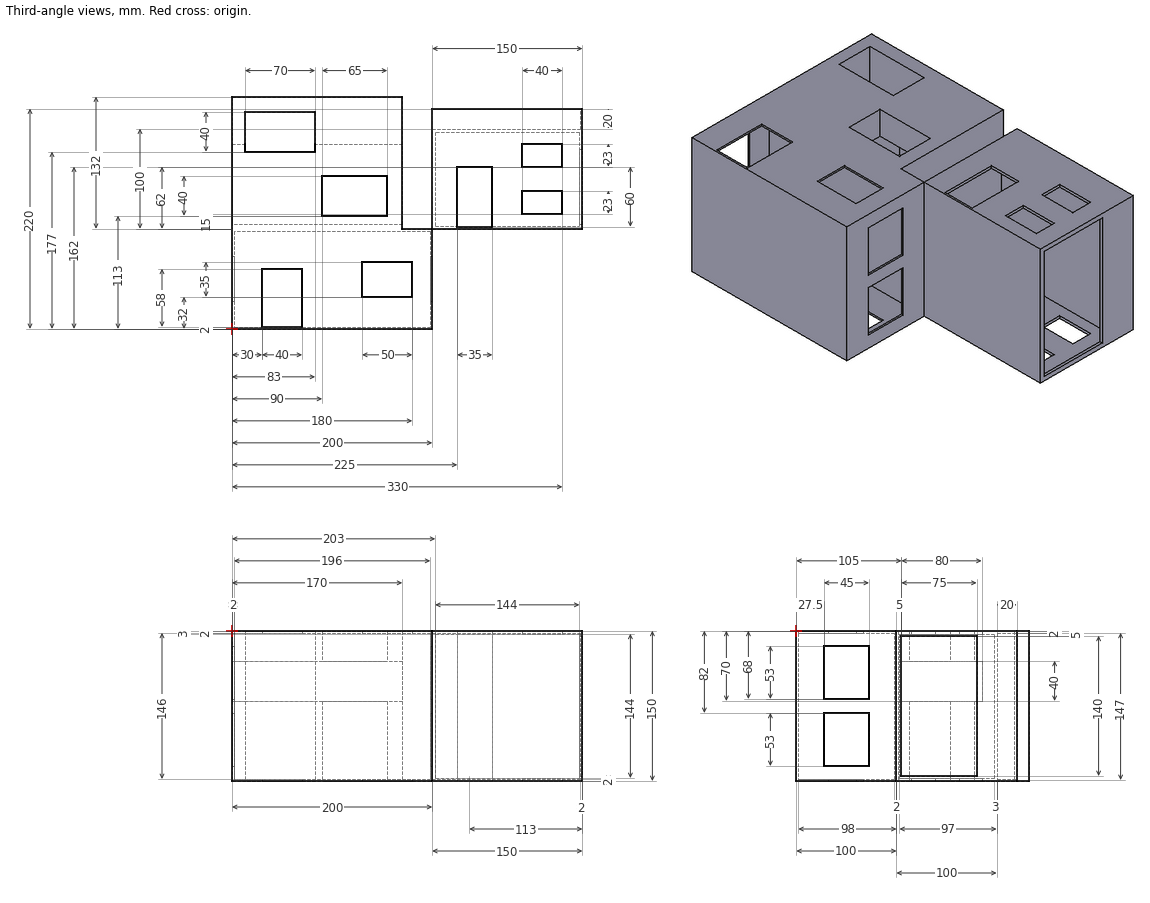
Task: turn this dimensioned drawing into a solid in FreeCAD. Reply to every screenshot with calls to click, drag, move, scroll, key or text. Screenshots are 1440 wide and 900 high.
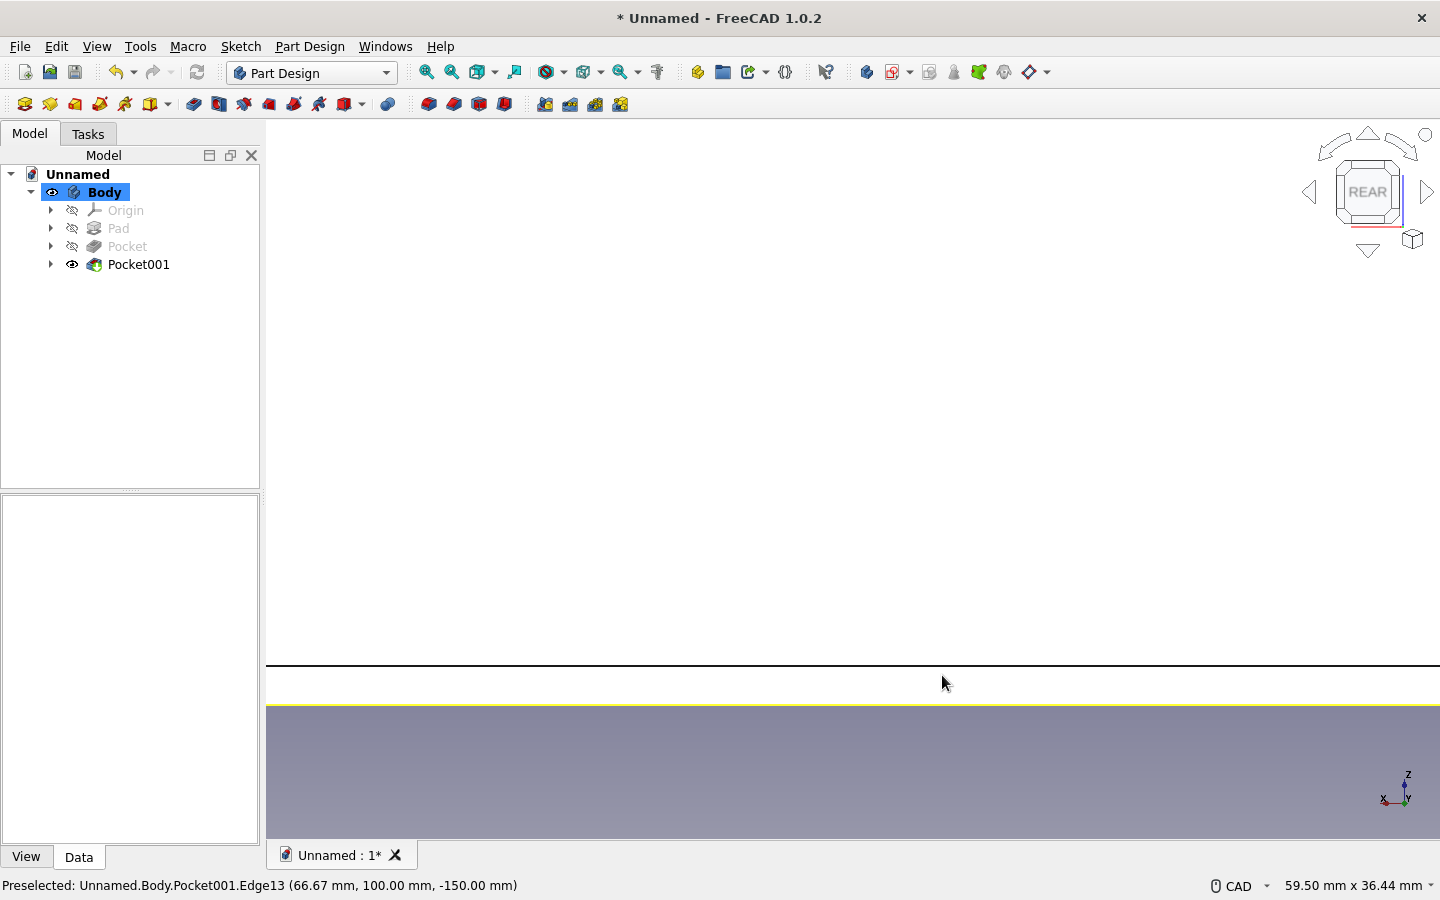
click(938, 678)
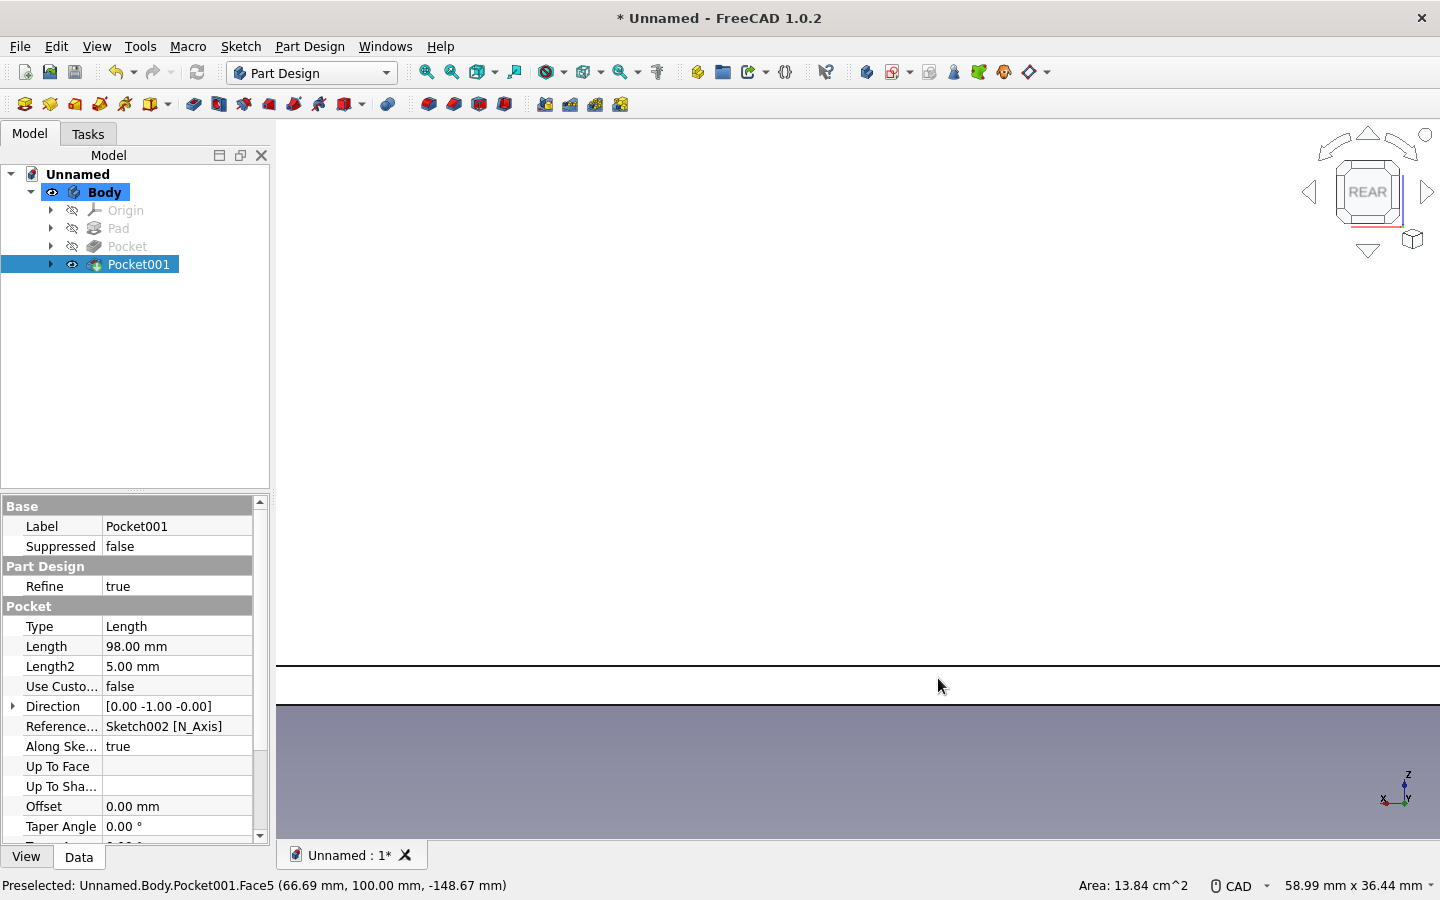
click(892, 72)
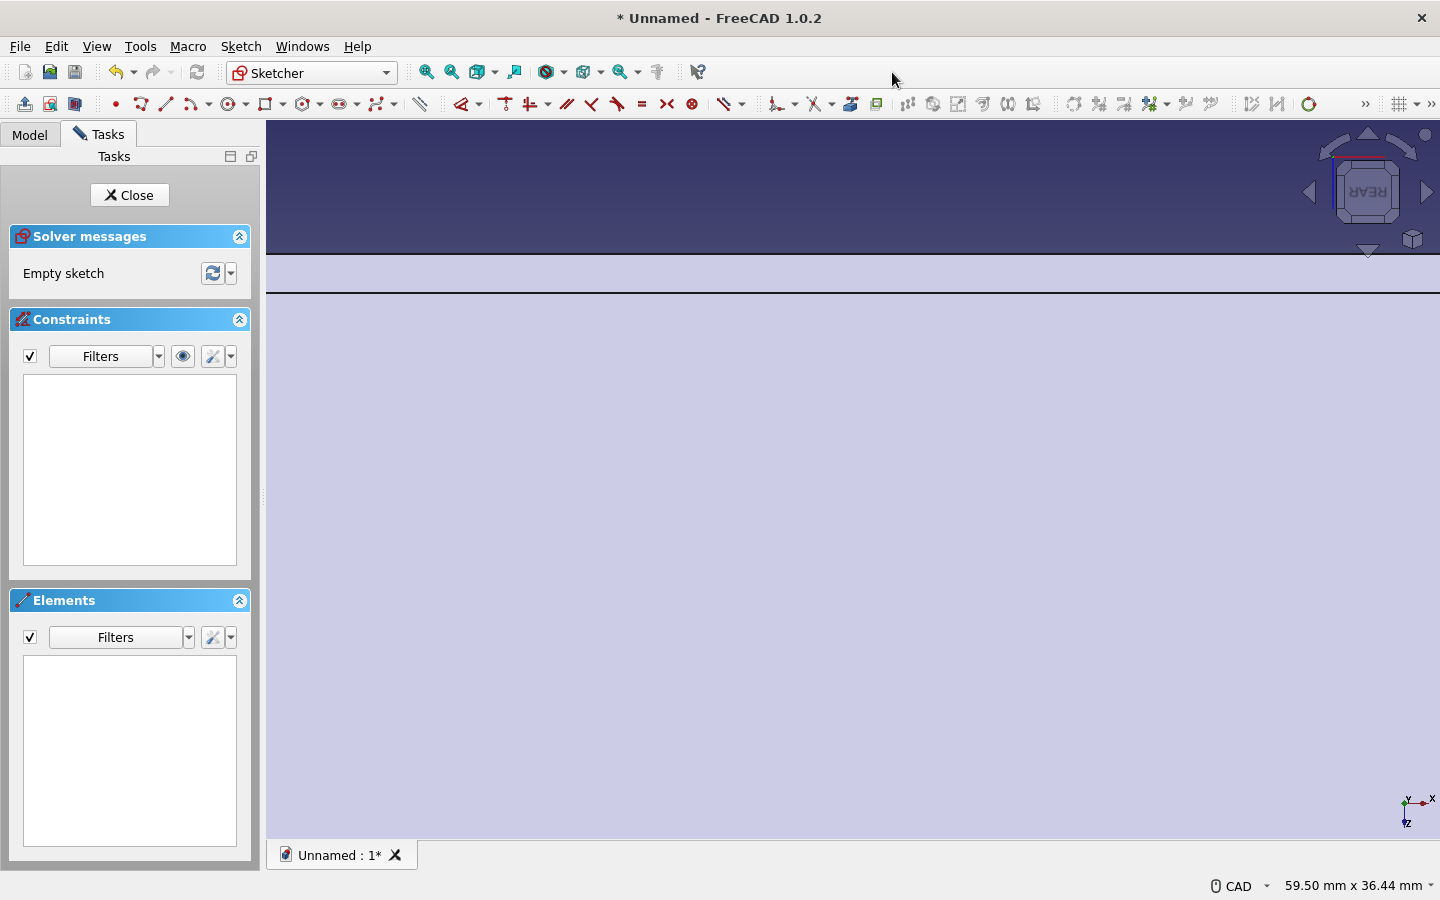
scroll(658, 231, down, 9)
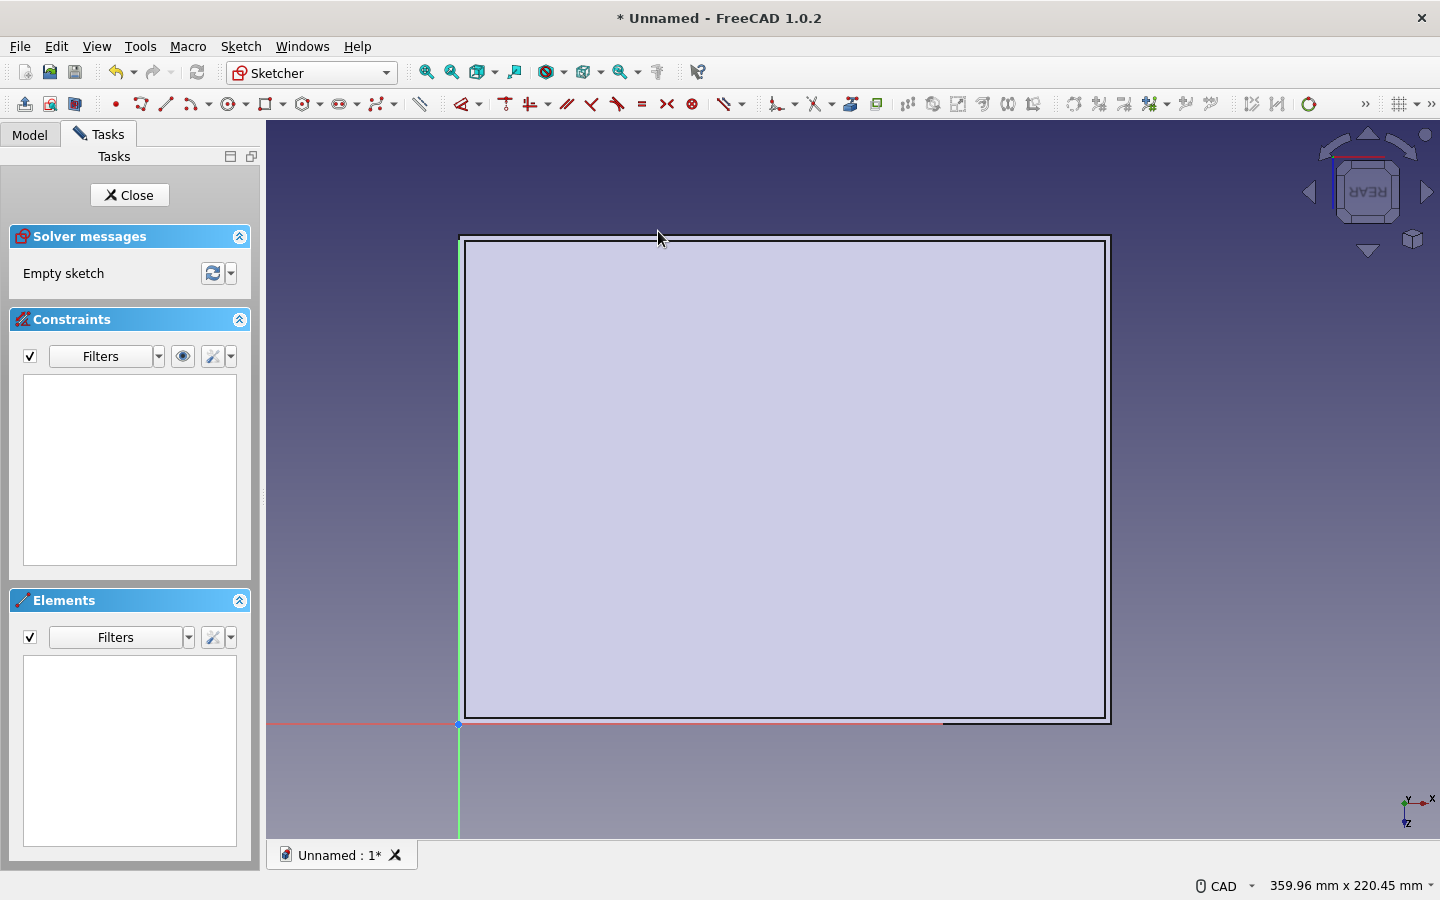
click(264, 104)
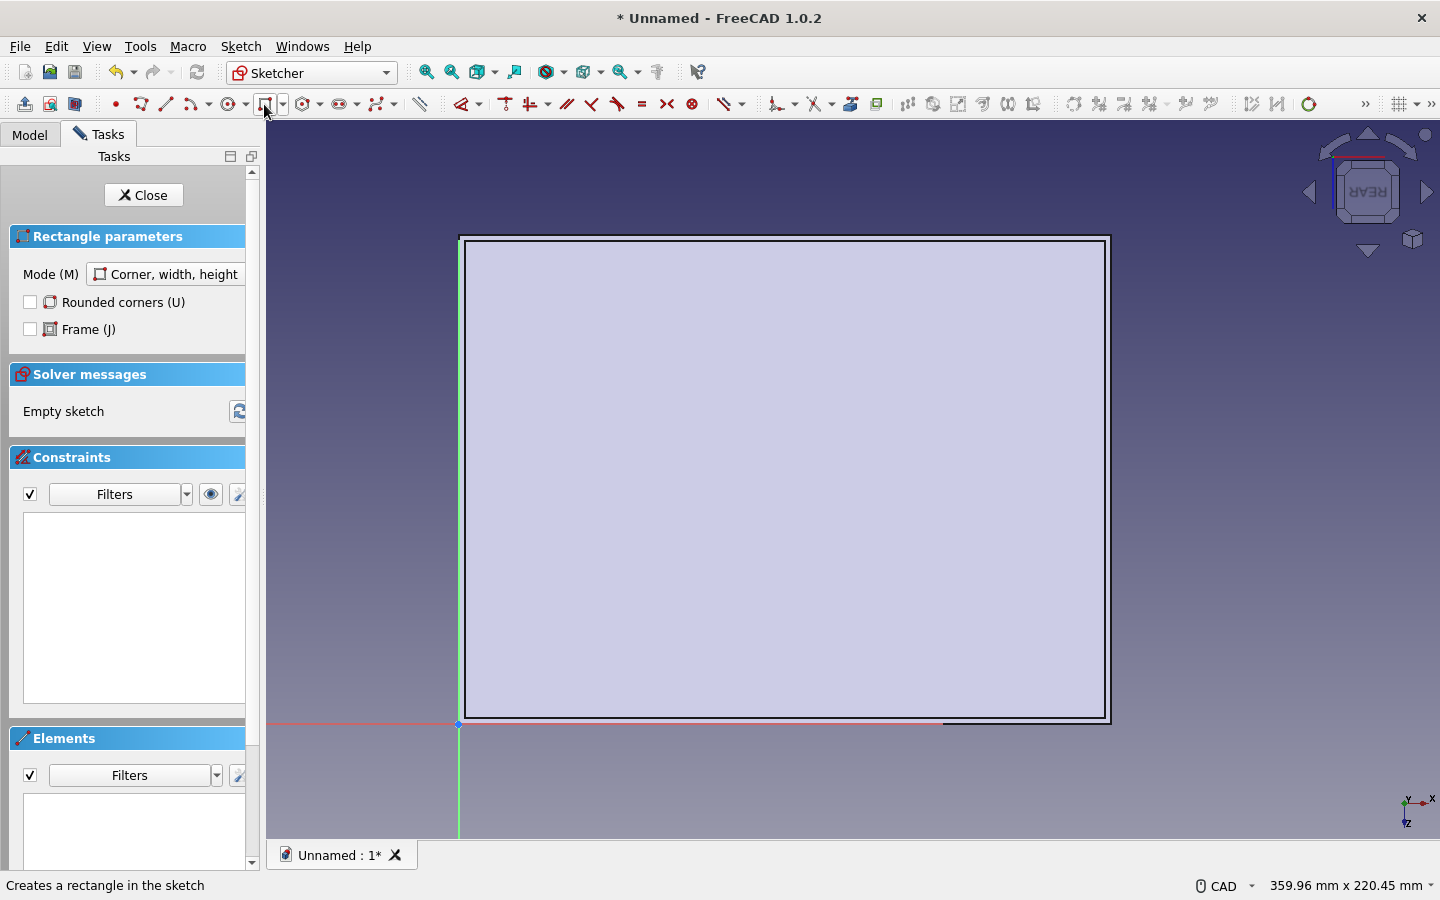
click(459, 724)
move(1111, 235)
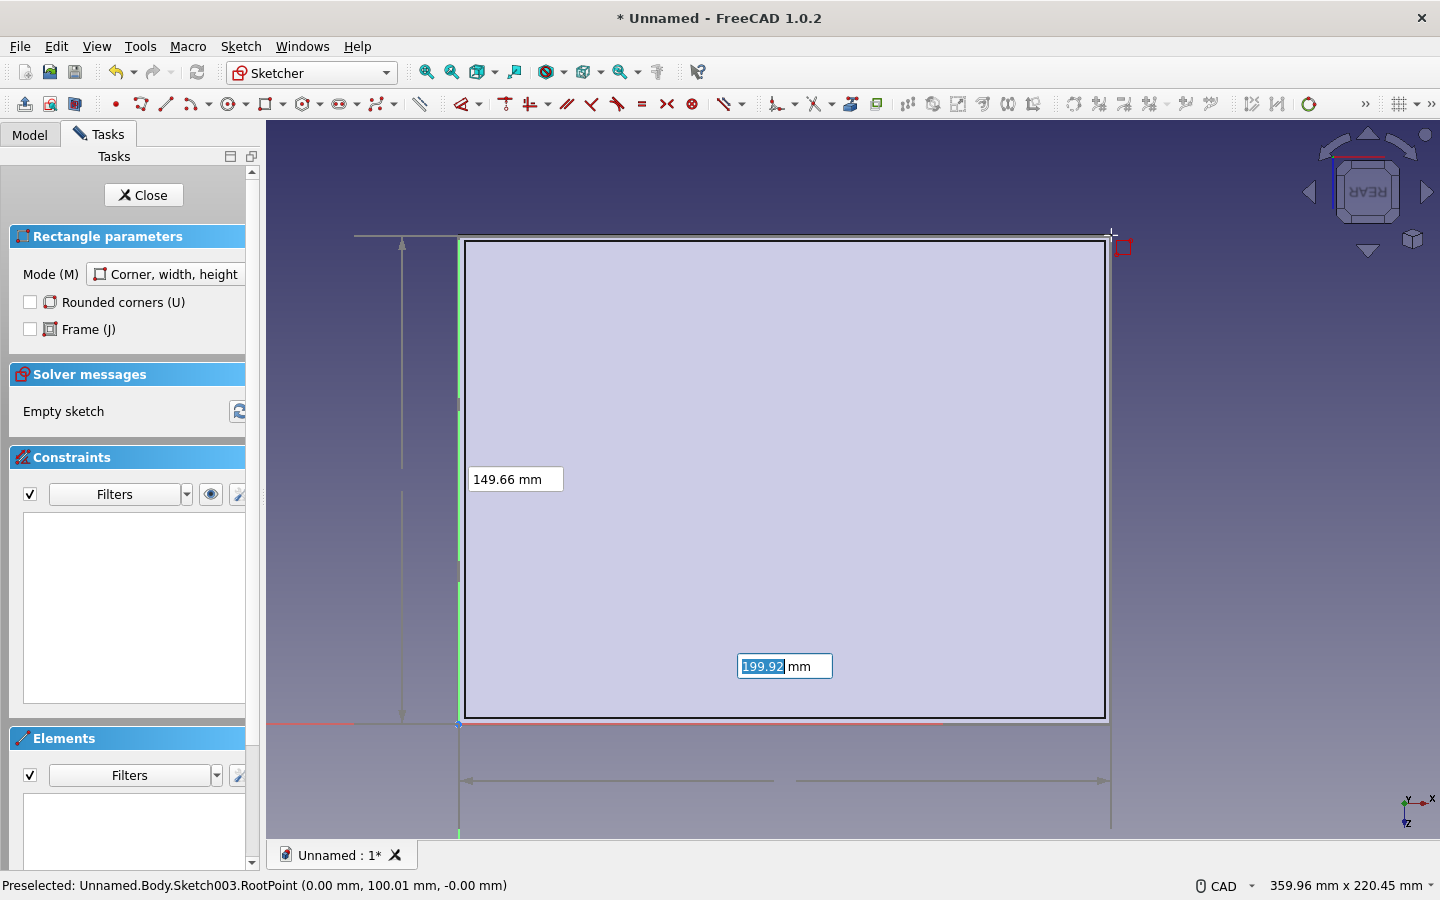
text(200)
key(Tab)
text(150)
key(Return)
key(Escape)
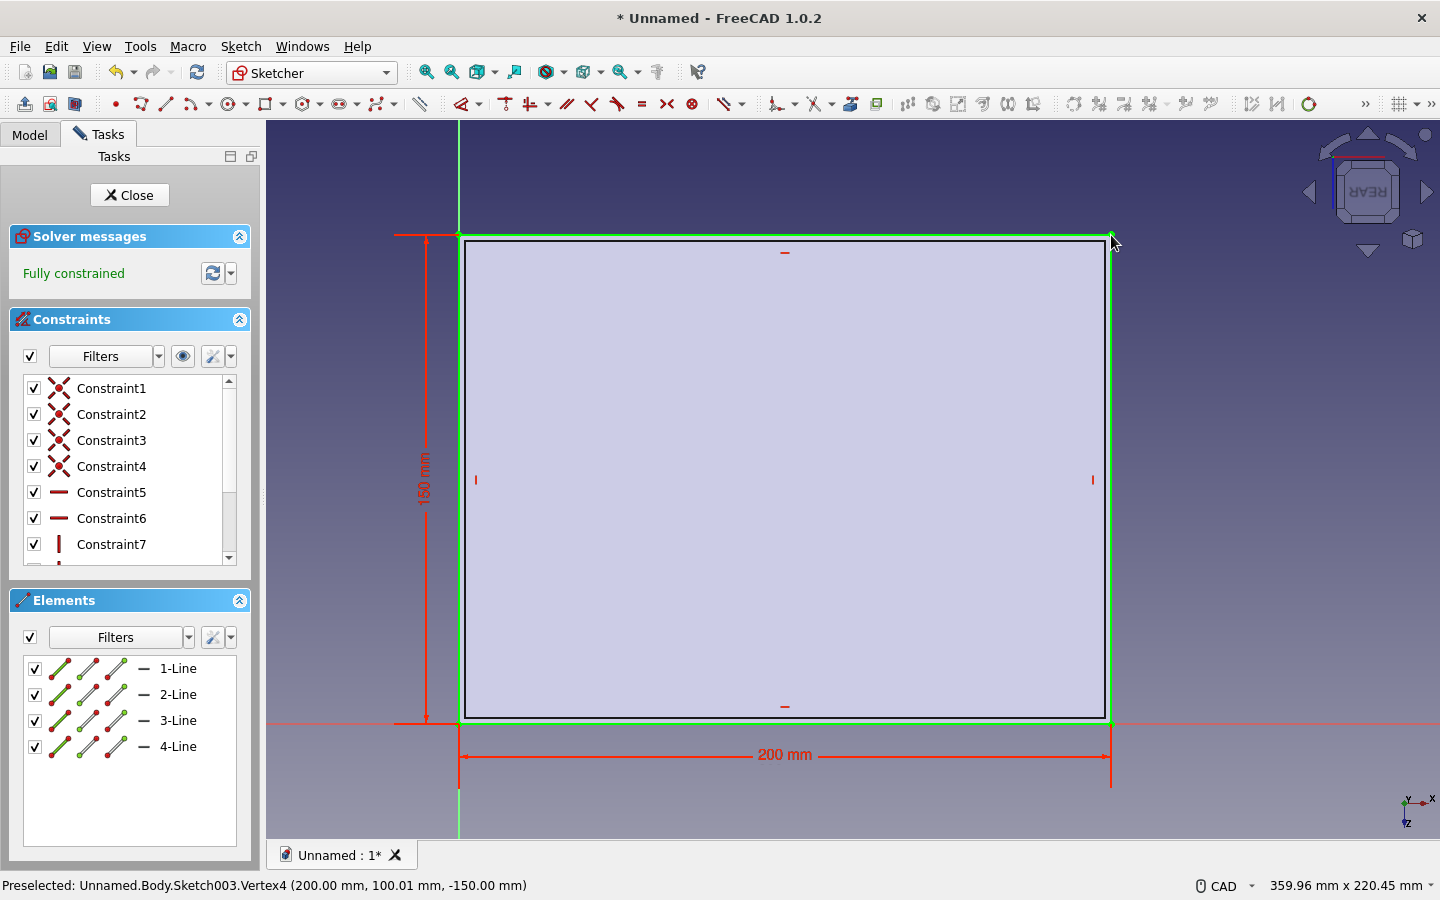
click(130, 195)